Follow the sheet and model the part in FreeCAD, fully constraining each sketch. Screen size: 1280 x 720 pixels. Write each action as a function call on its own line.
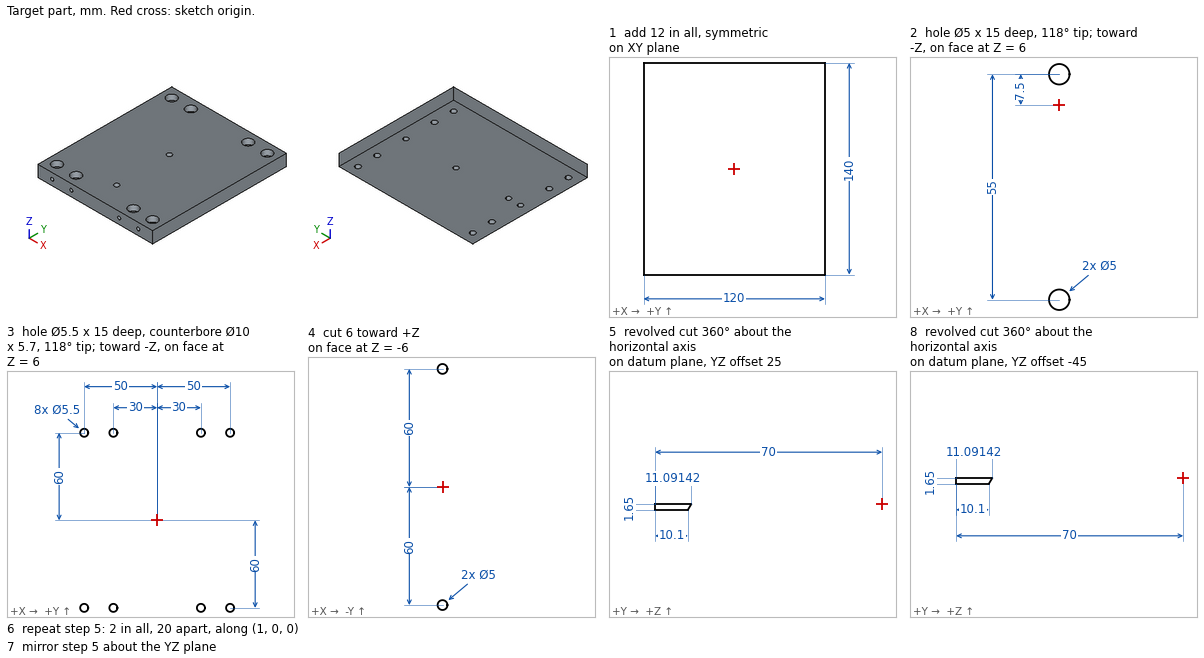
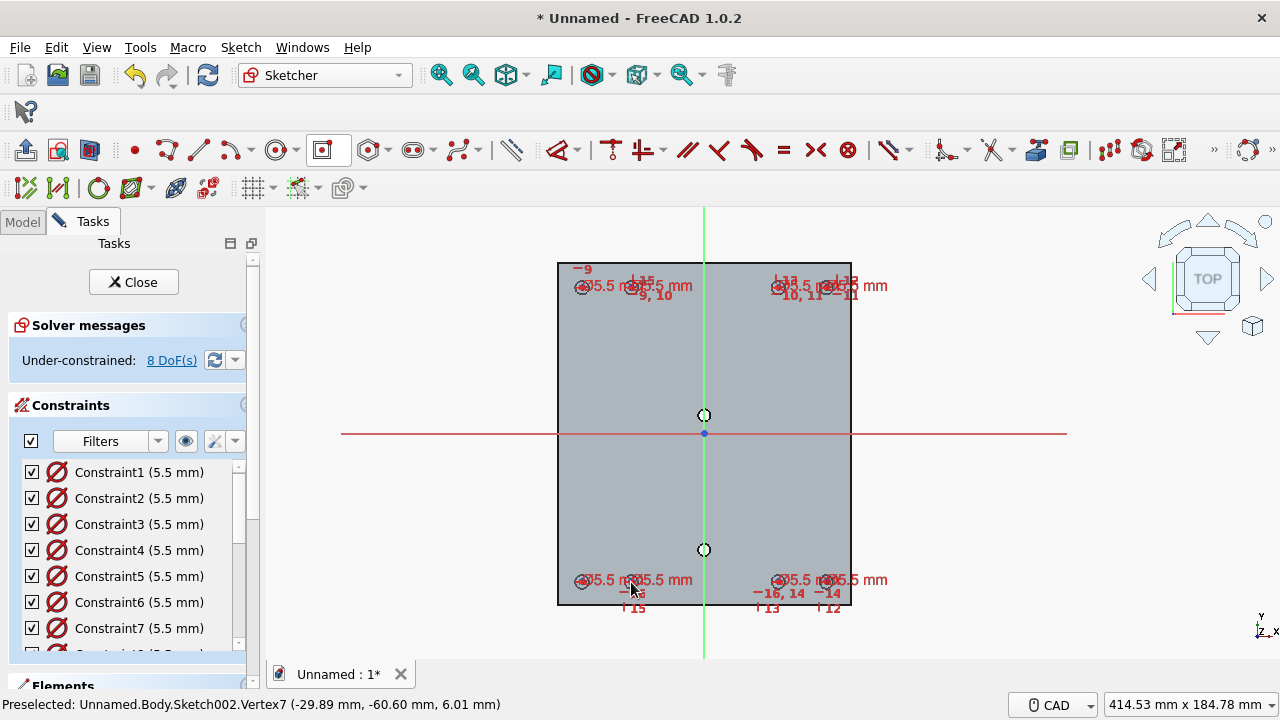
click(582, 288)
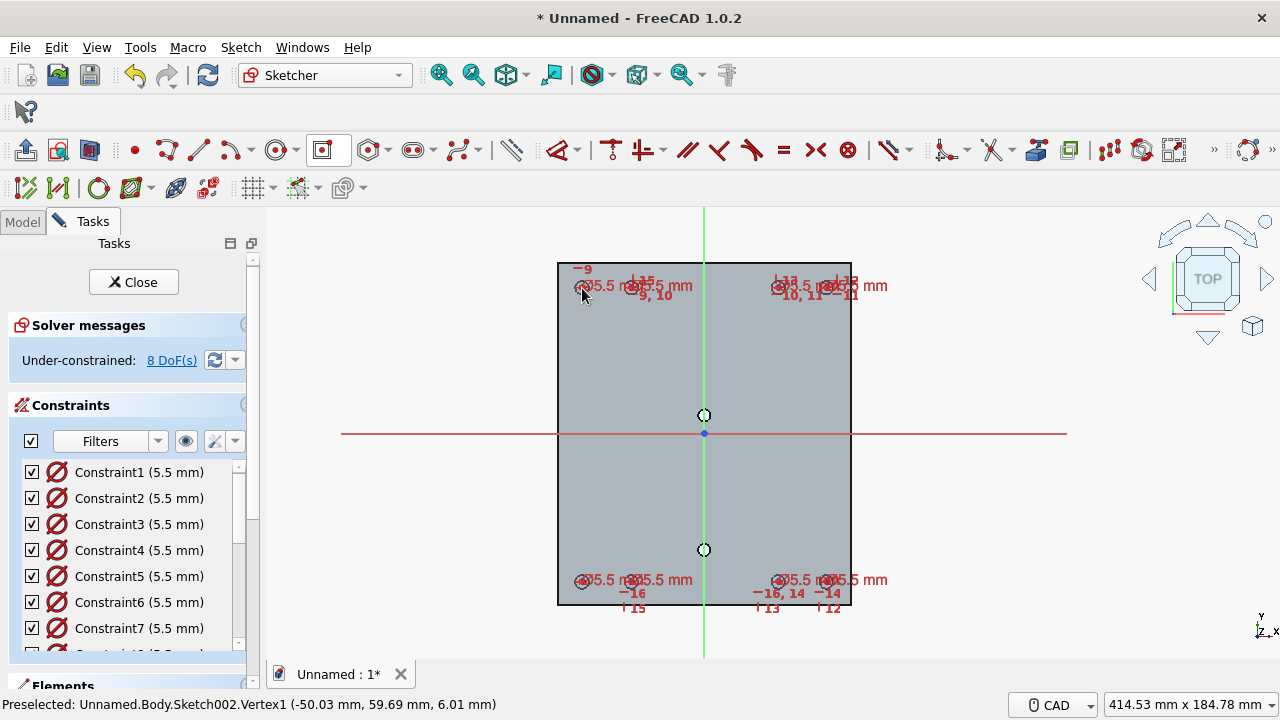
click(582, 582)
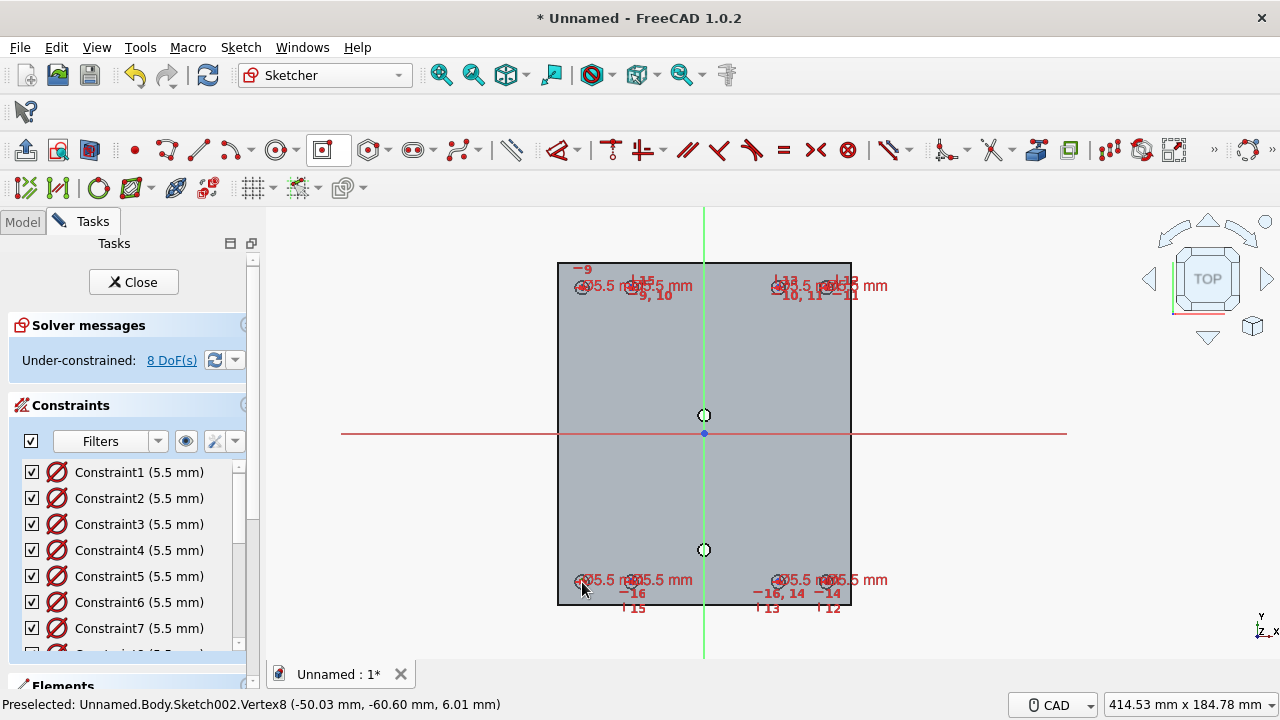
key(v)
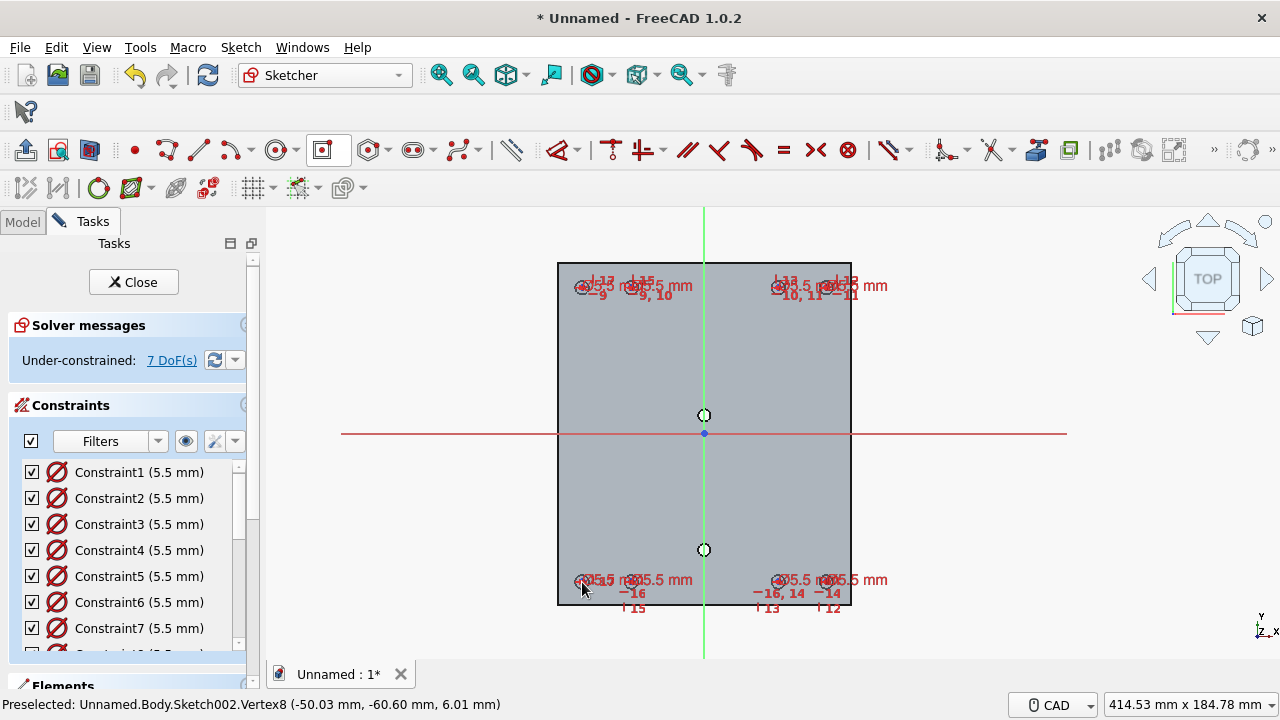
click(631, 582)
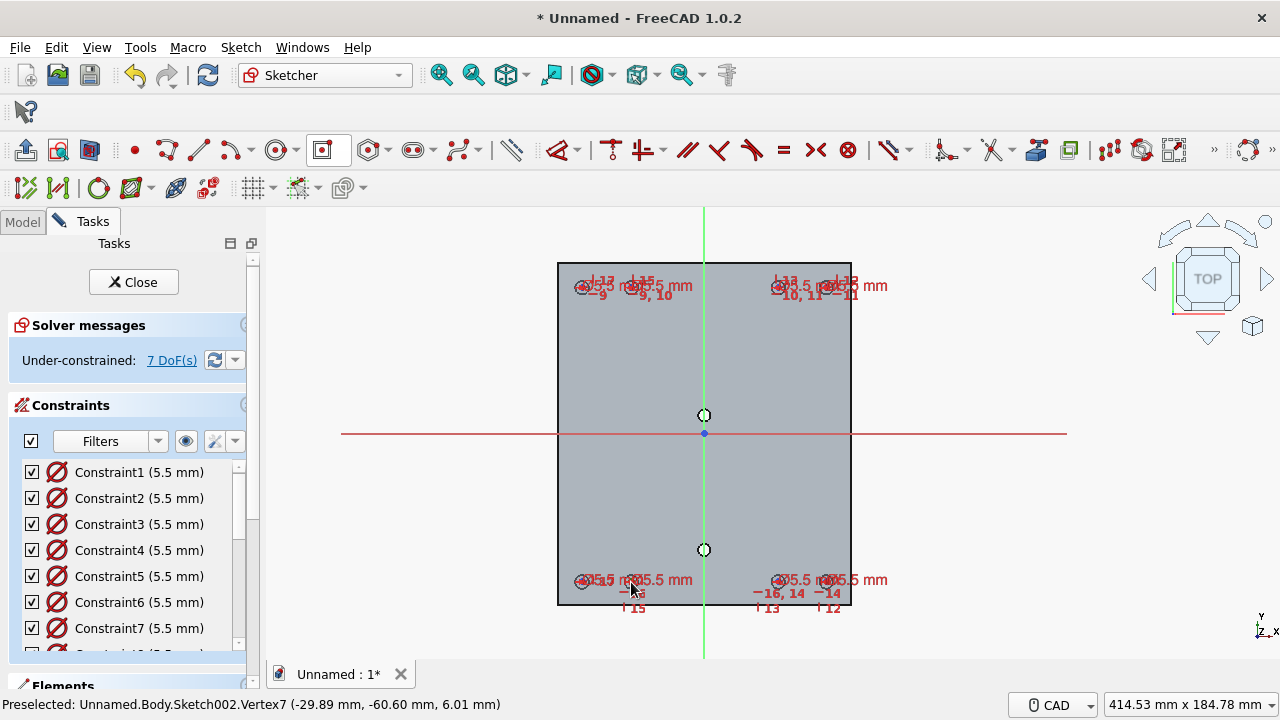
click(582, 582)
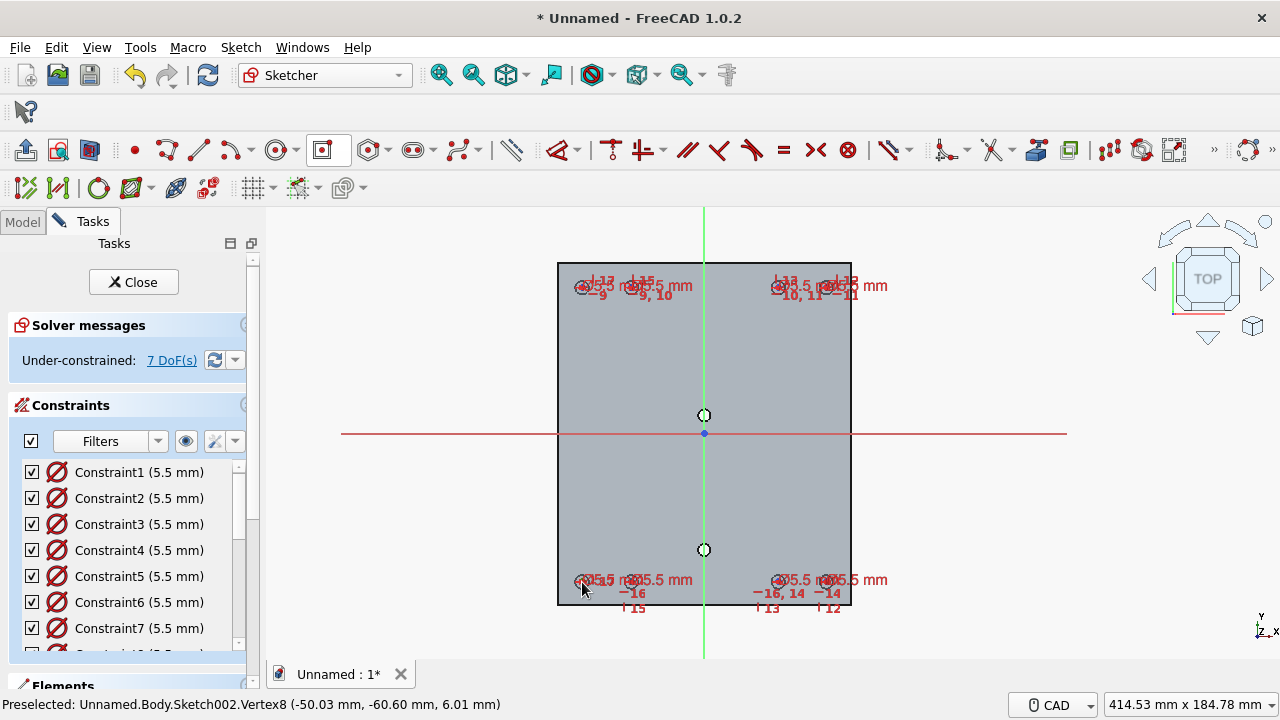
key(h)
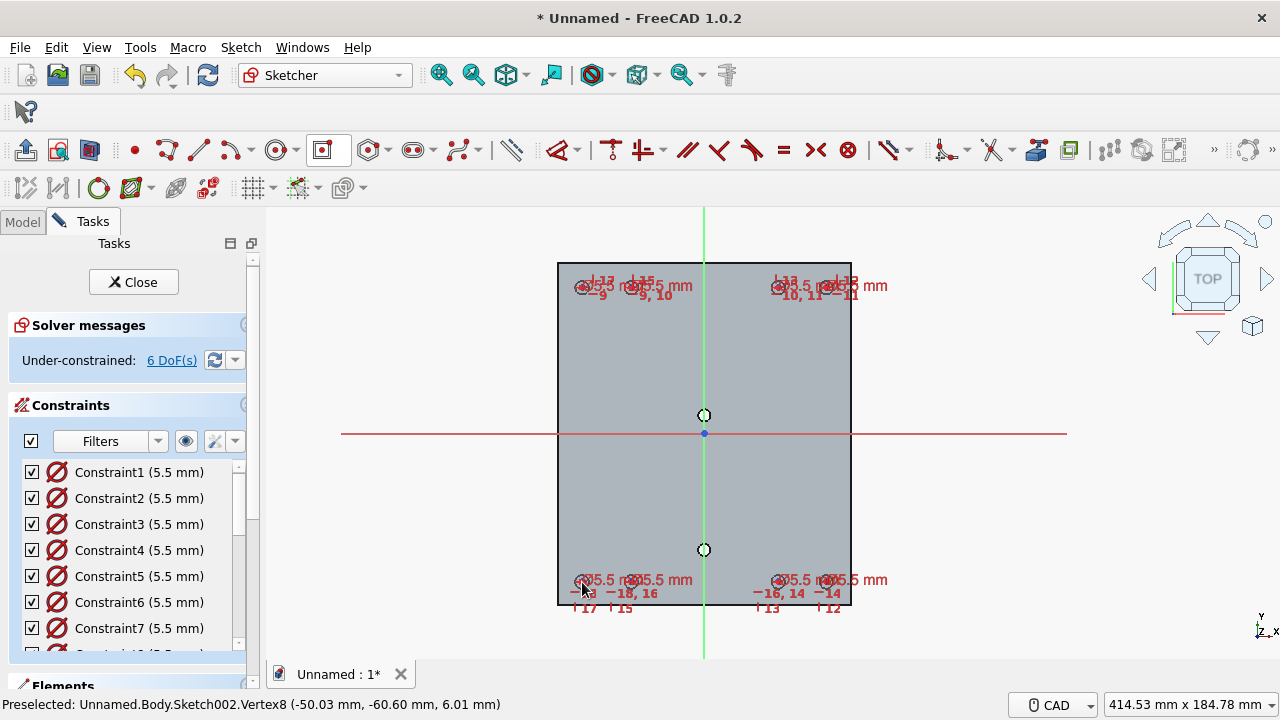
click(558, 150)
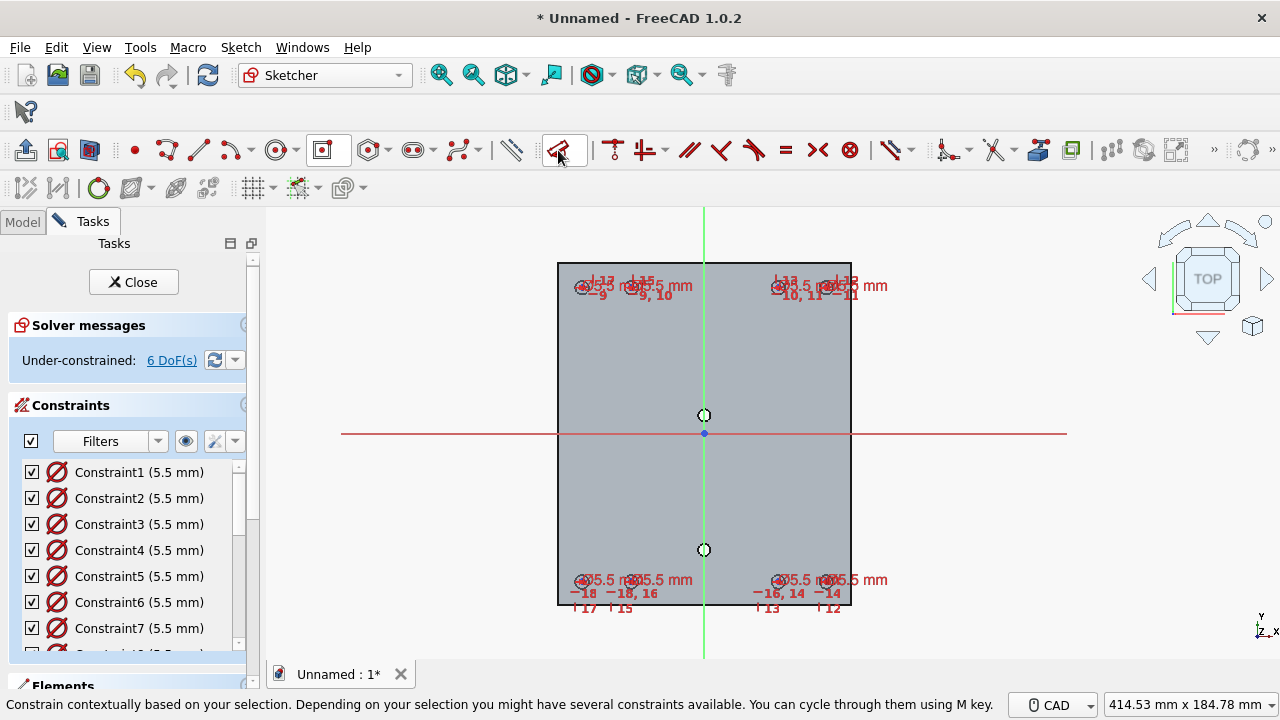
click(582, 288)
click(643, 254)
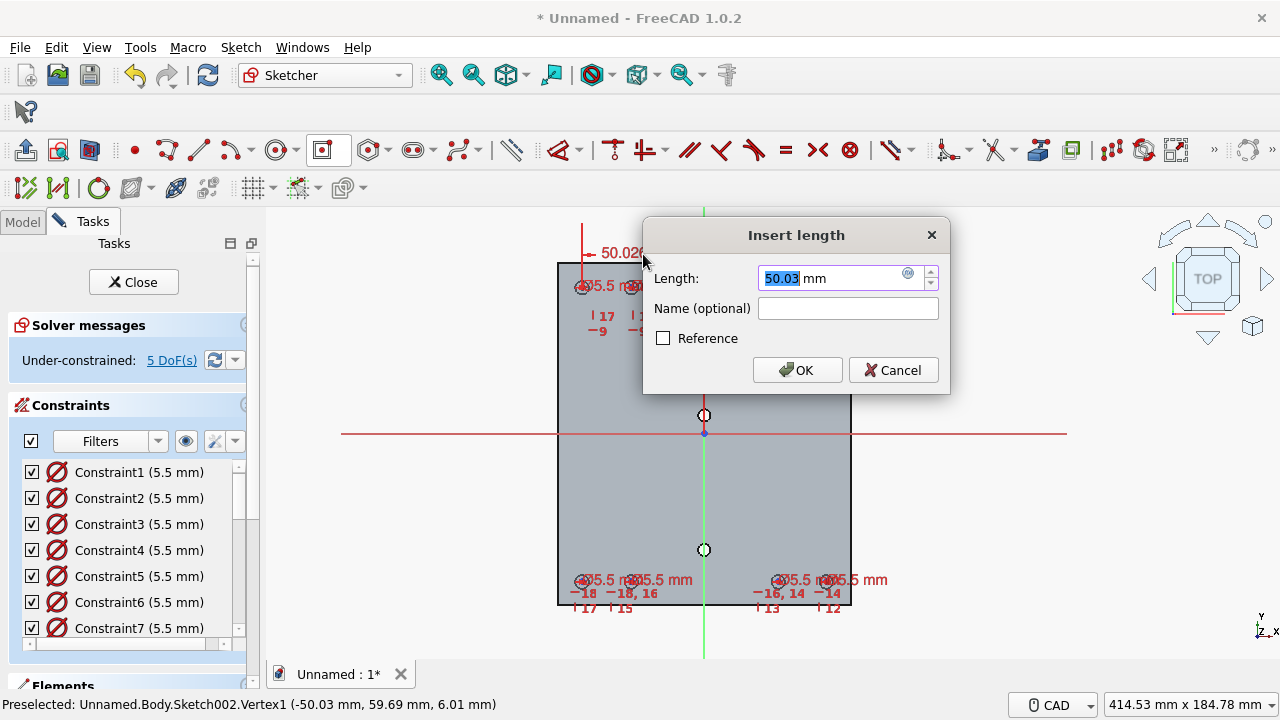
text(50)
key(Return)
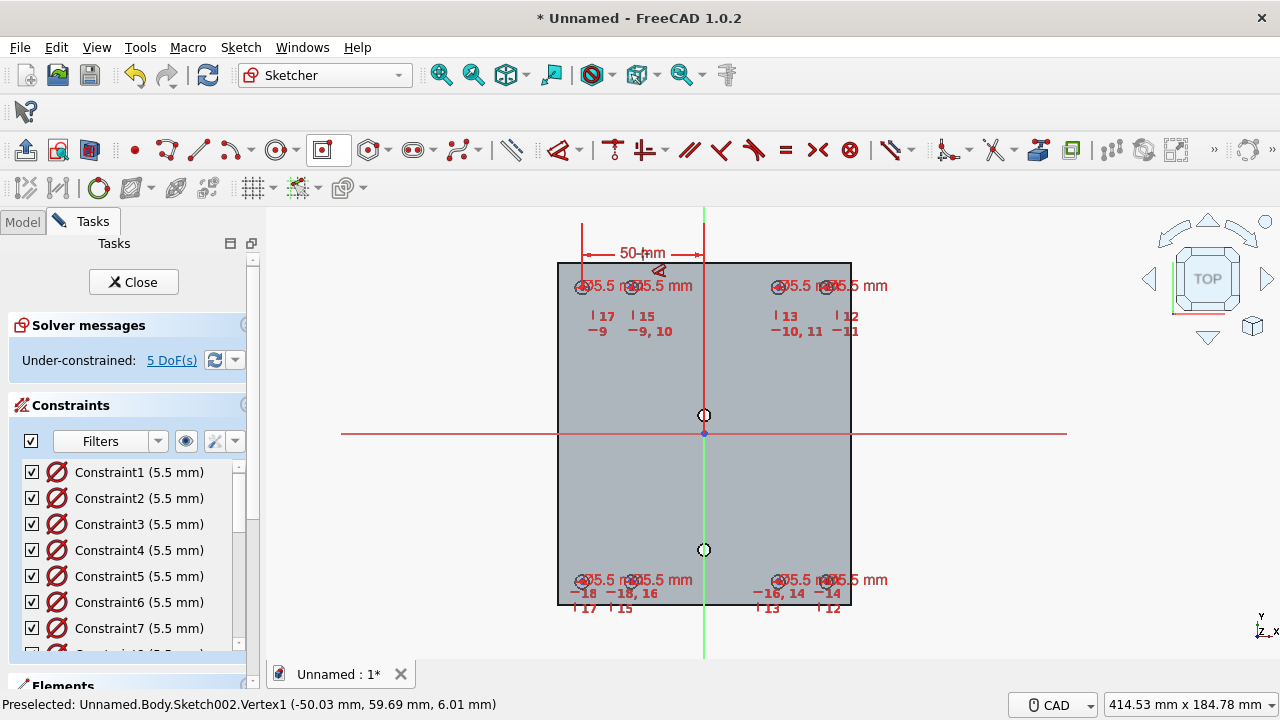
click(582, 288)
click(548, 361)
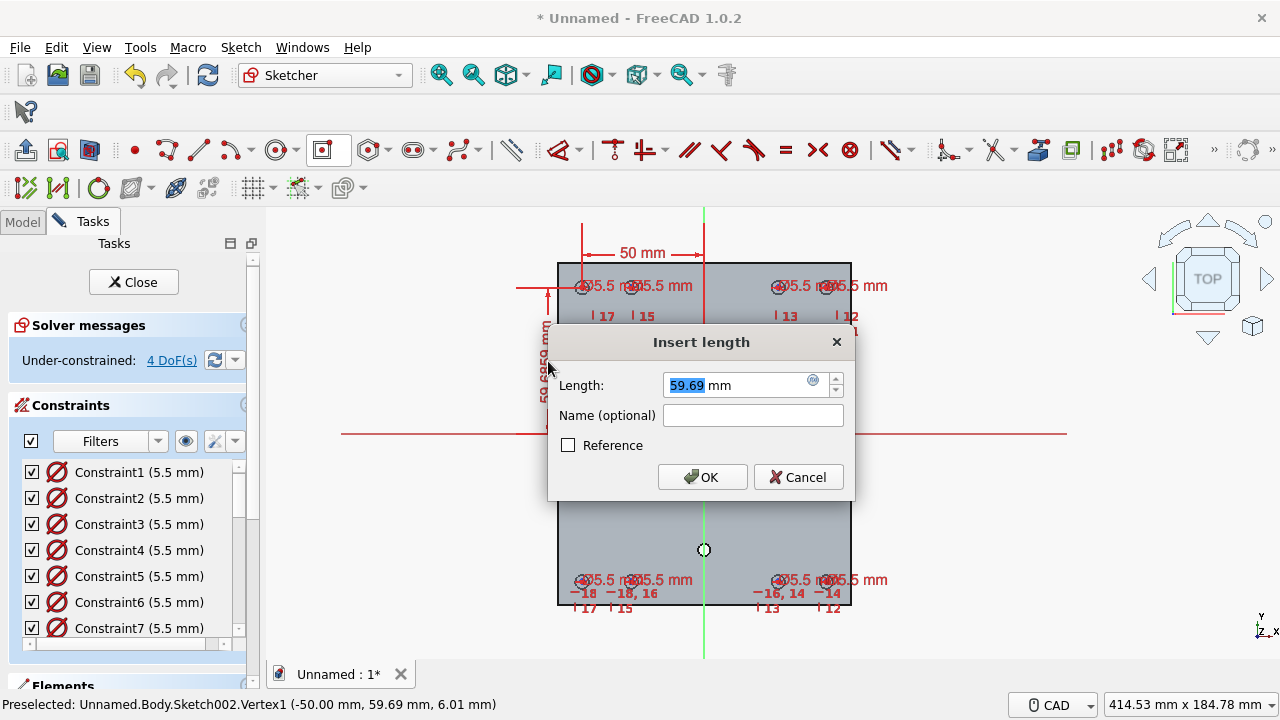
text(60)
key(Return)